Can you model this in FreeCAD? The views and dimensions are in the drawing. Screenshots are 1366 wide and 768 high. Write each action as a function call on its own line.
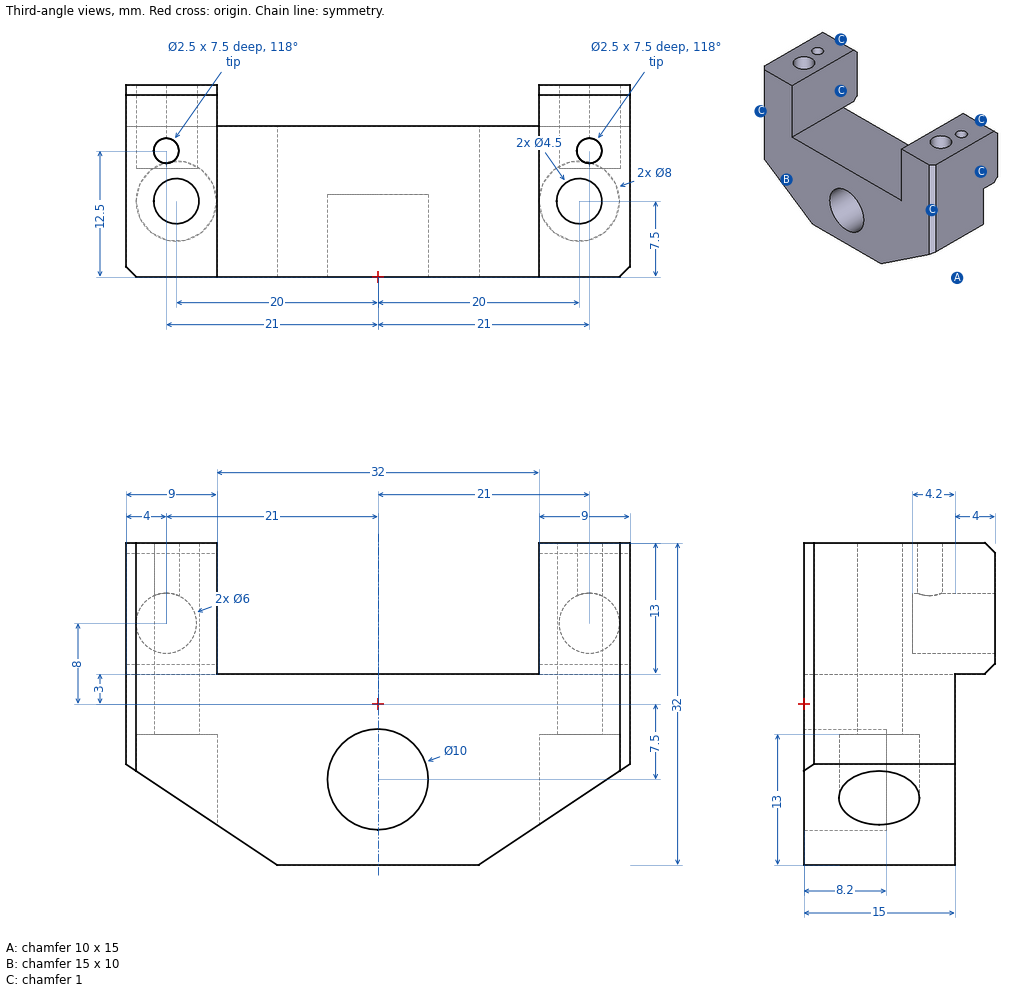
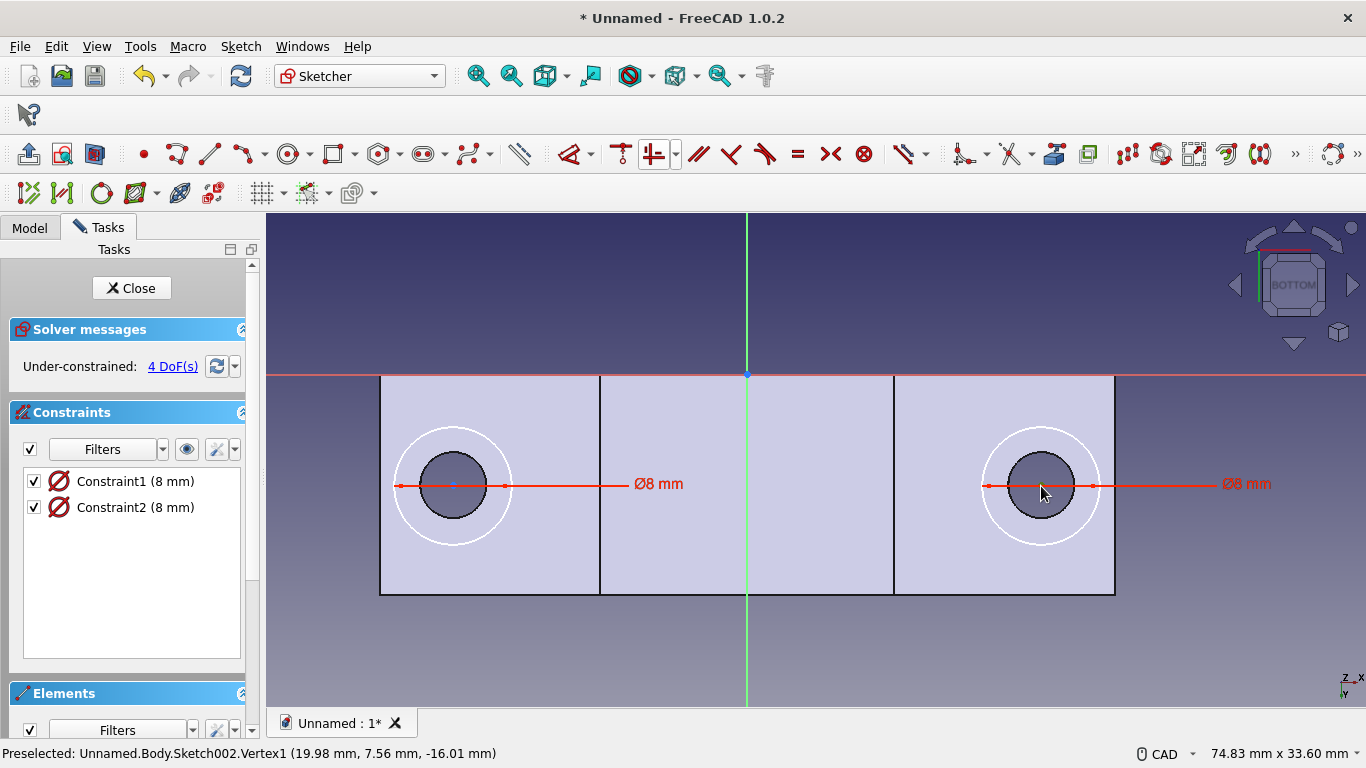
click(453, 486)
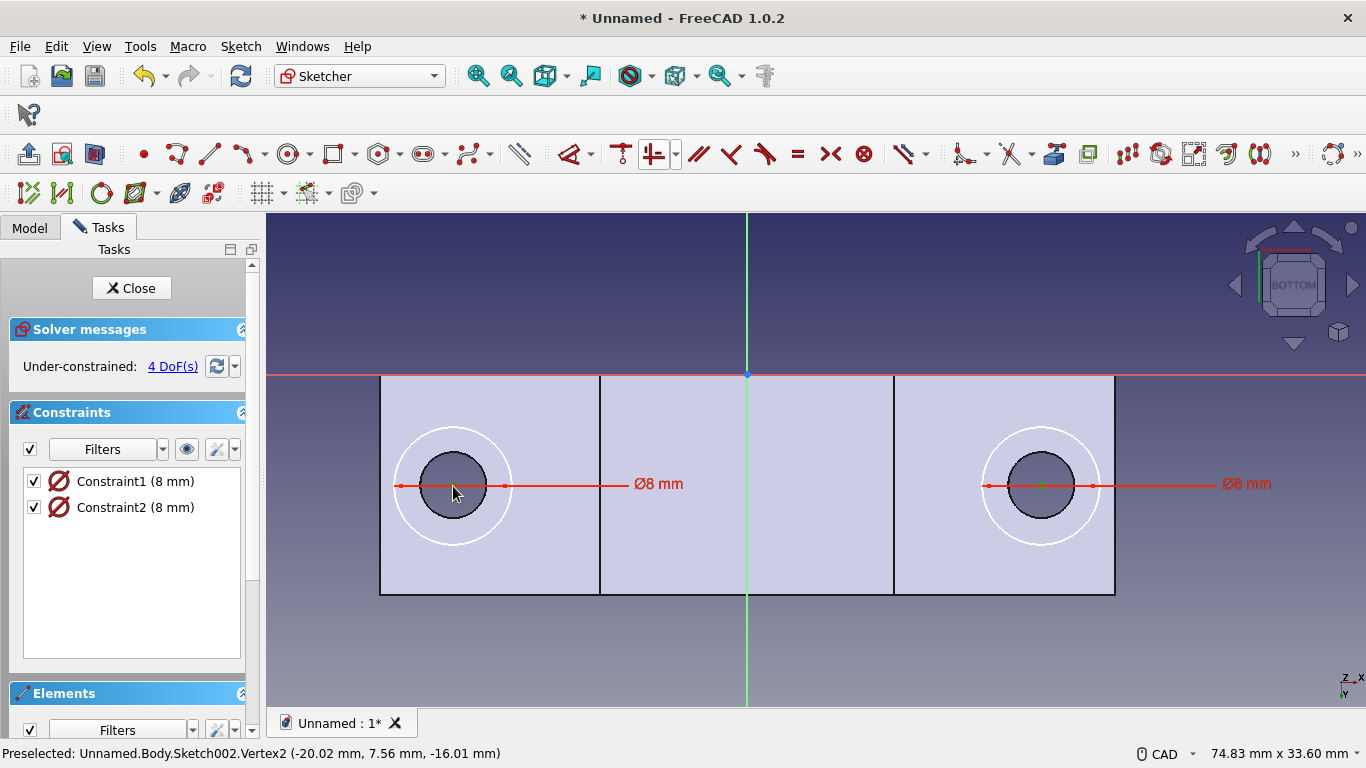
key(h)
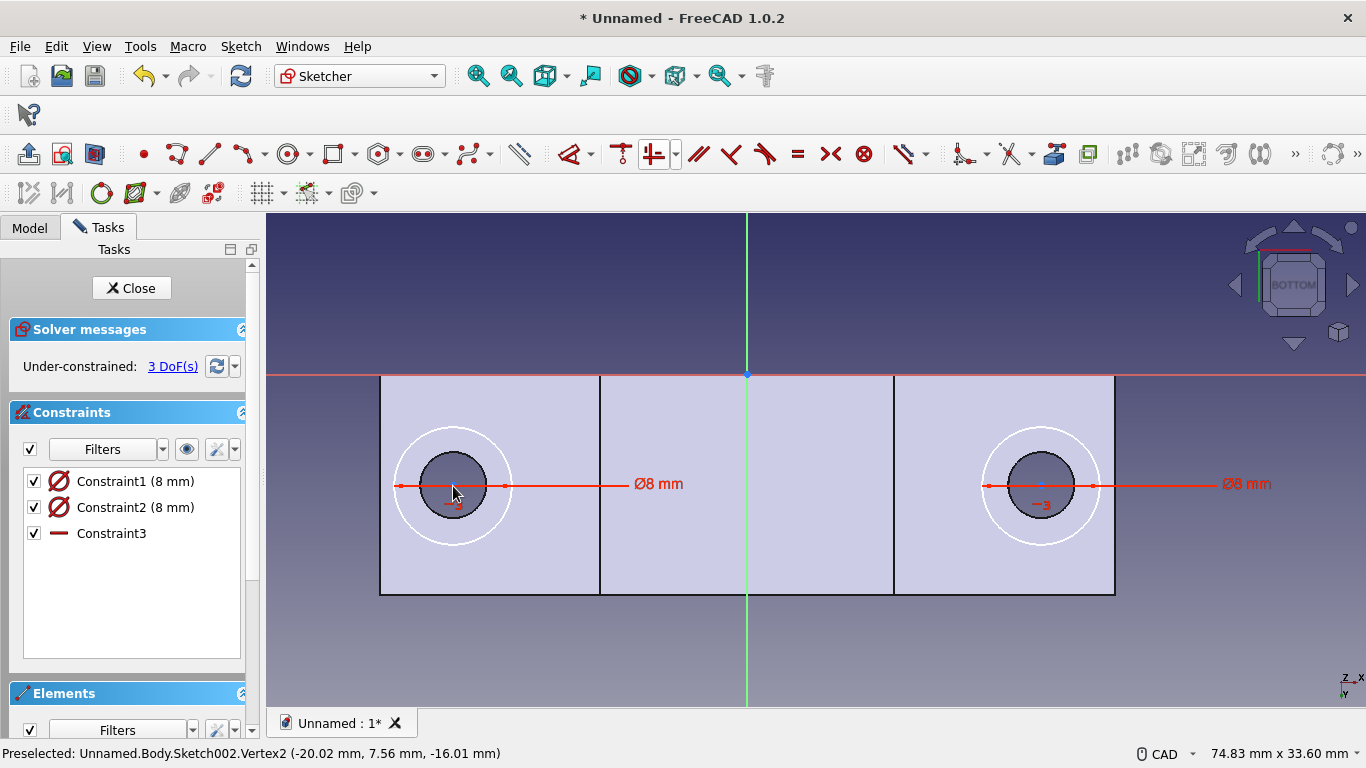
click(568, 154)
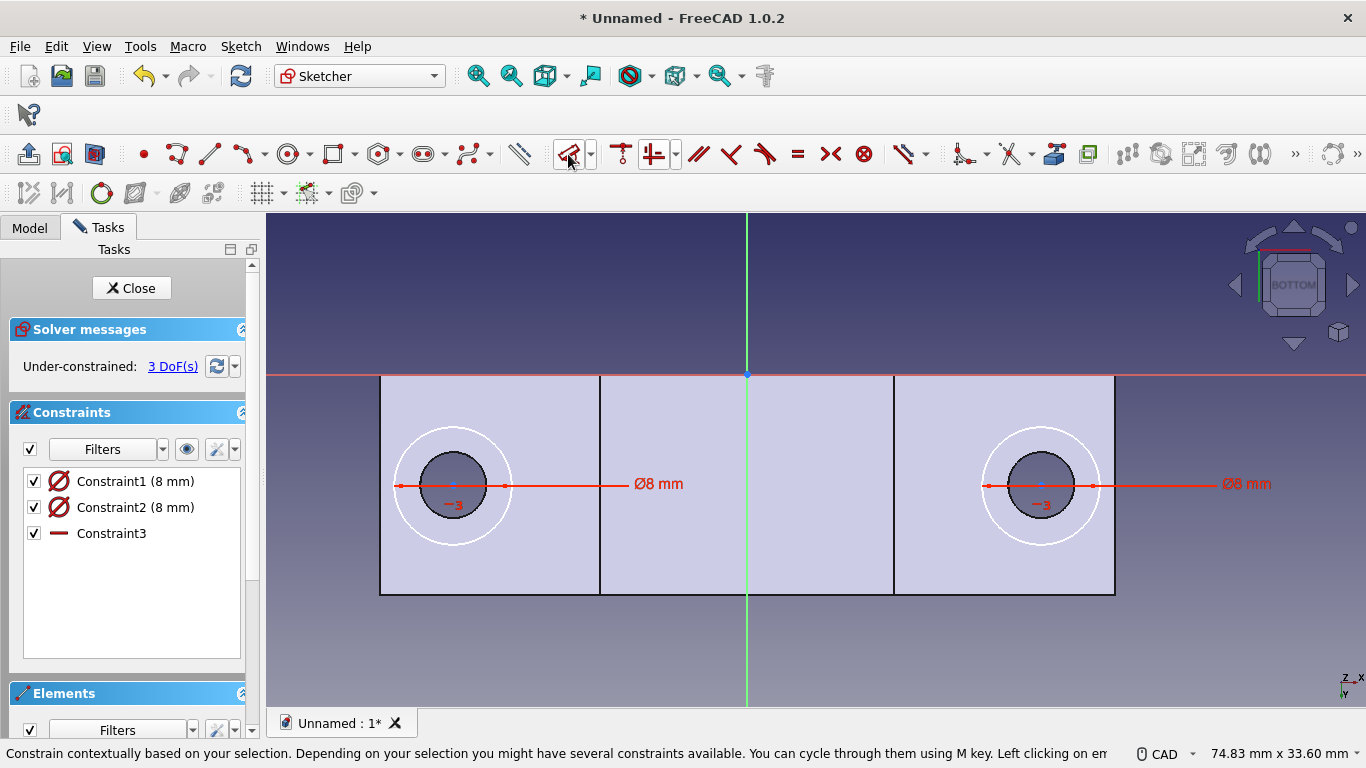
click(1041, 486)
click(894, 341)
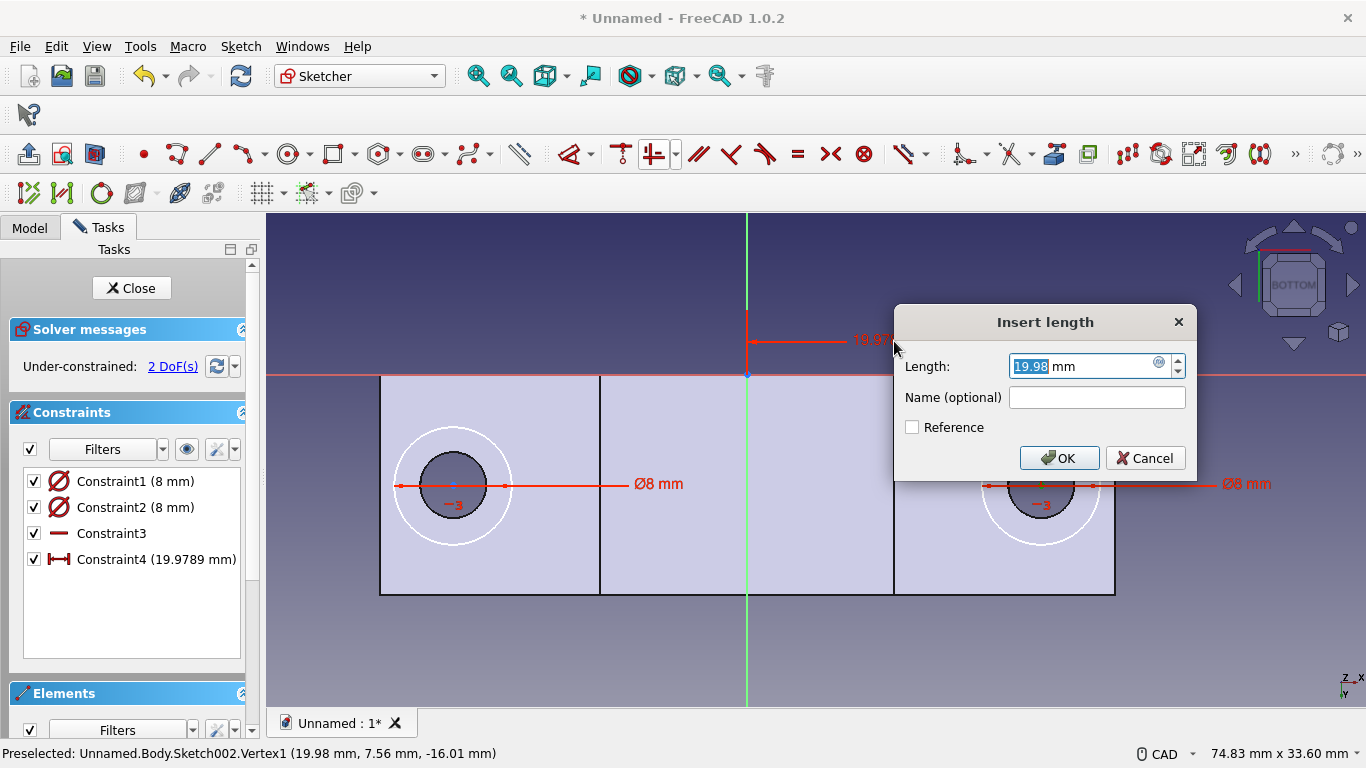
text(20)
key(Return)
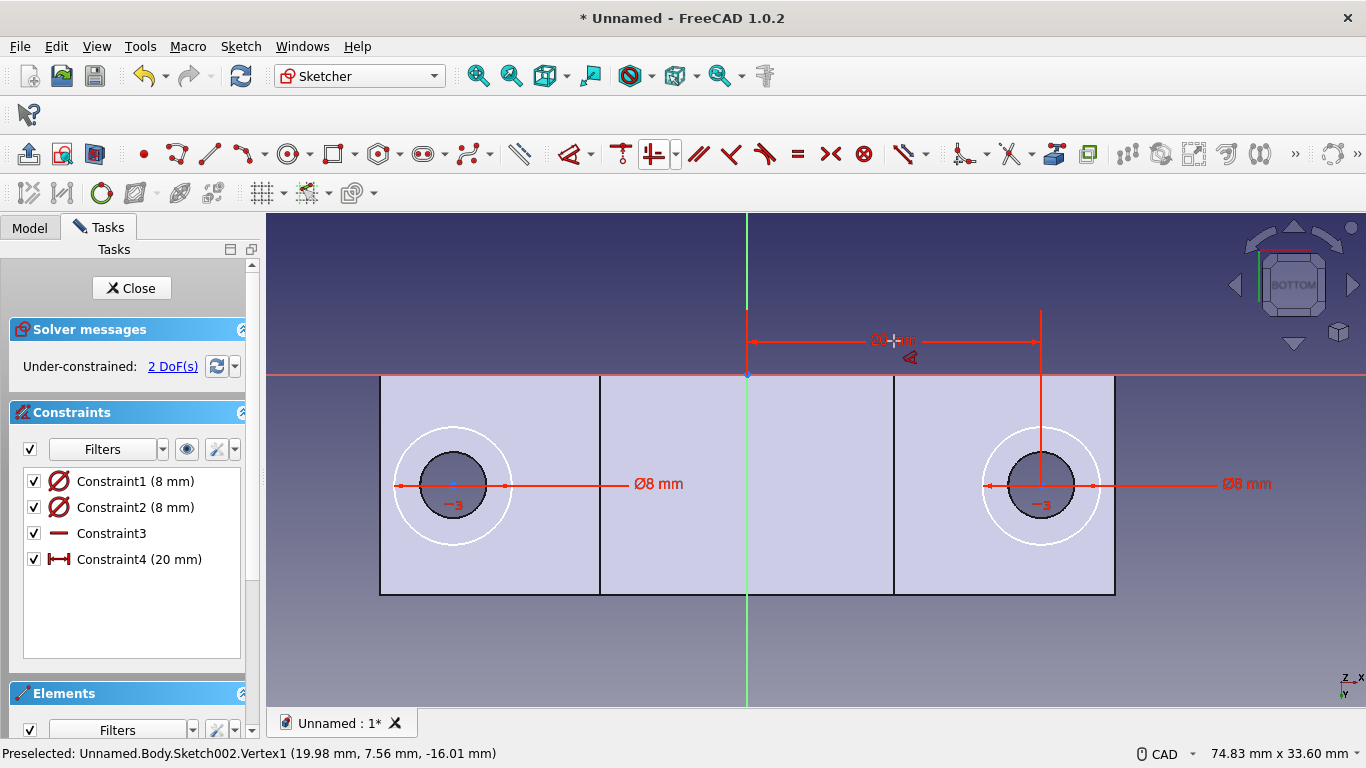
click(453, 486)
click(600, 341)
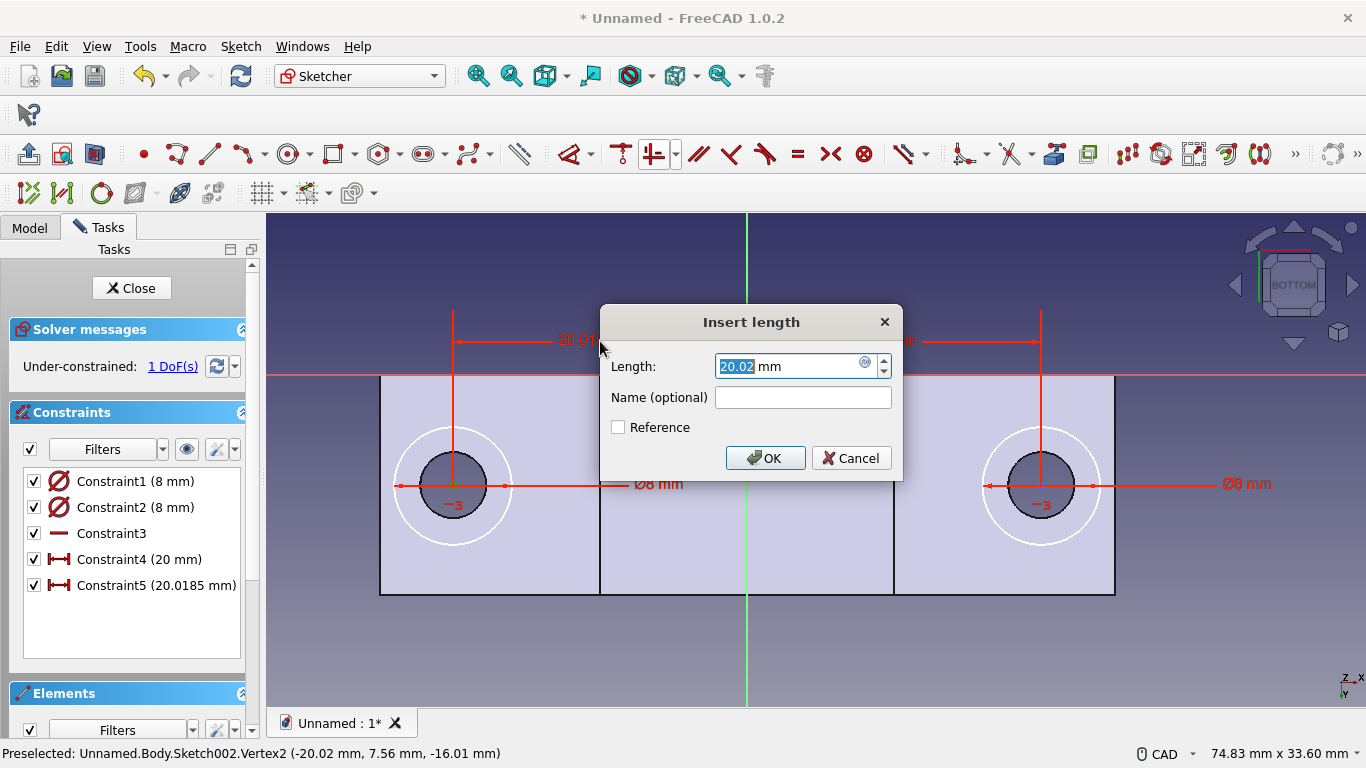
text(20)
key(Return)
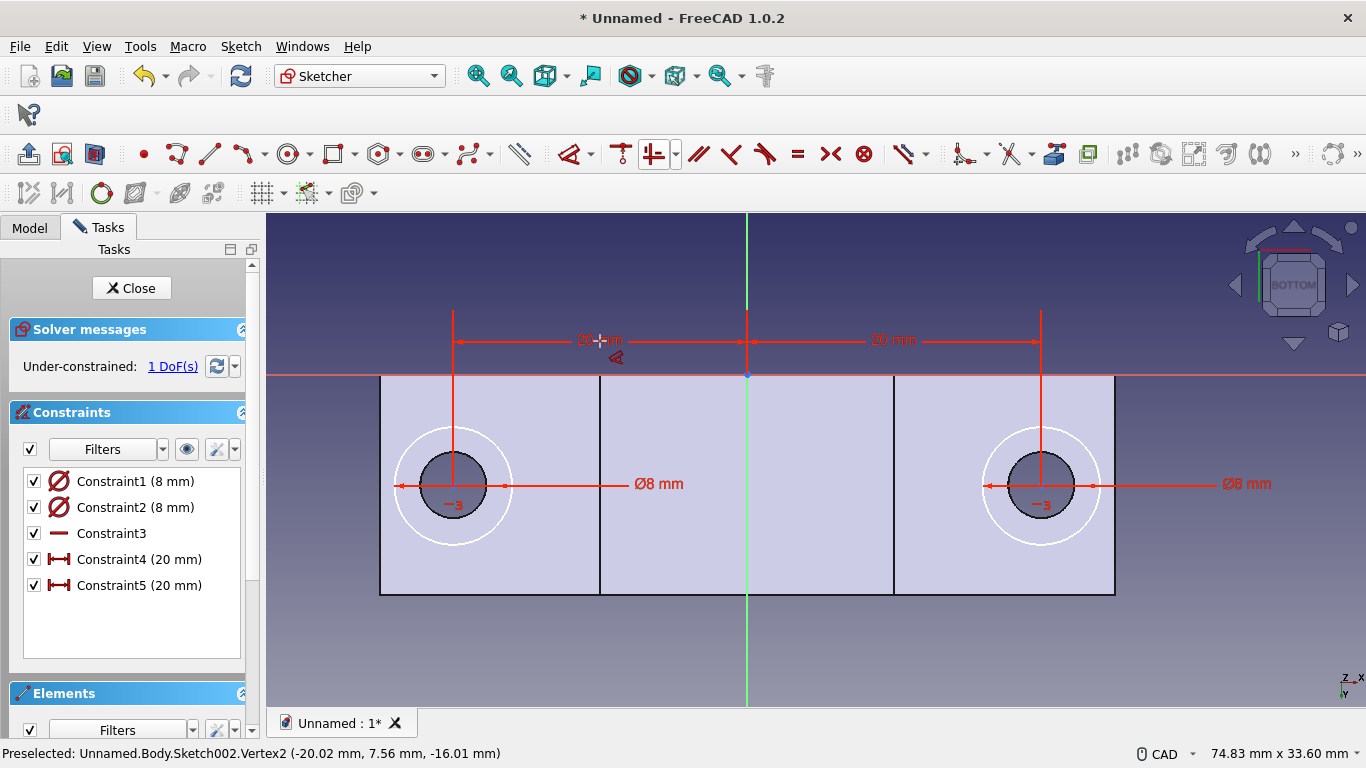
click(1041, 486)
click(1075, 405)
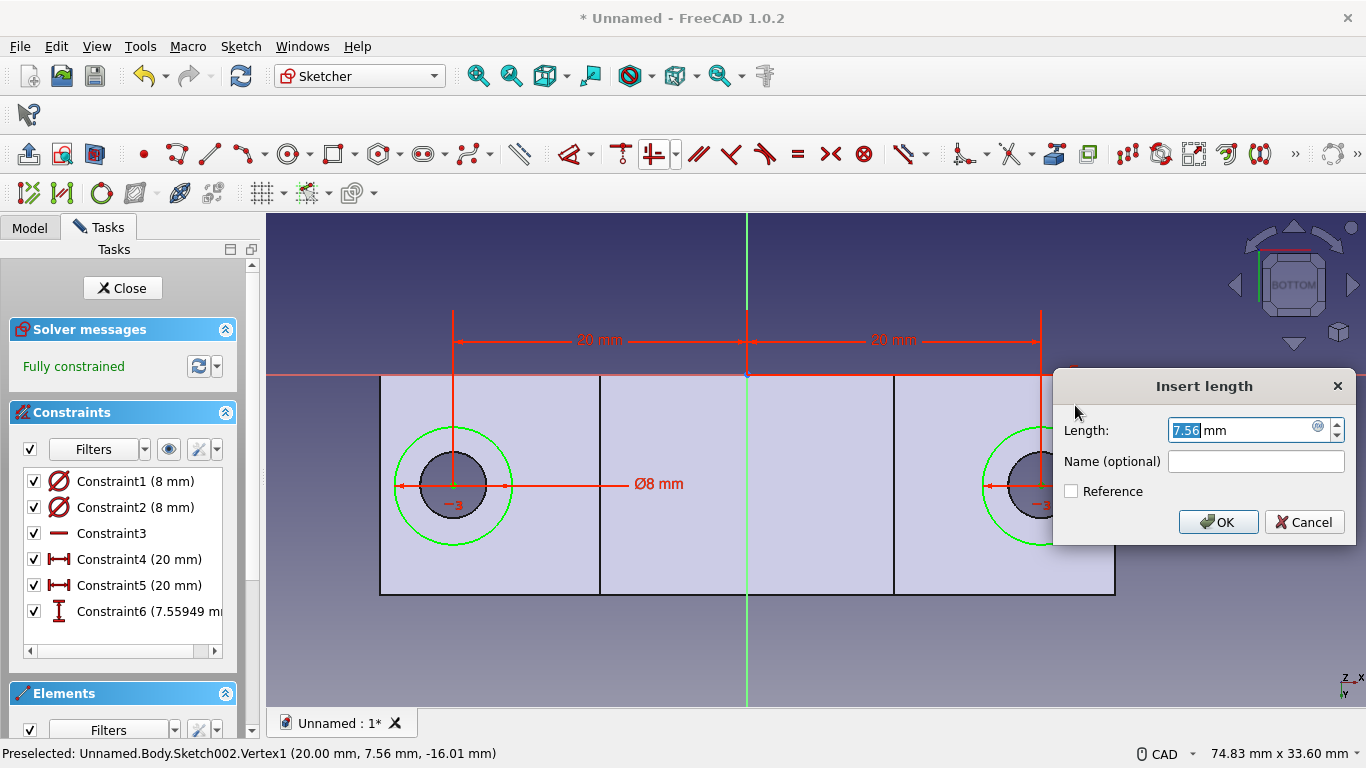
text(7.5)
key(Return)
key(Escape)